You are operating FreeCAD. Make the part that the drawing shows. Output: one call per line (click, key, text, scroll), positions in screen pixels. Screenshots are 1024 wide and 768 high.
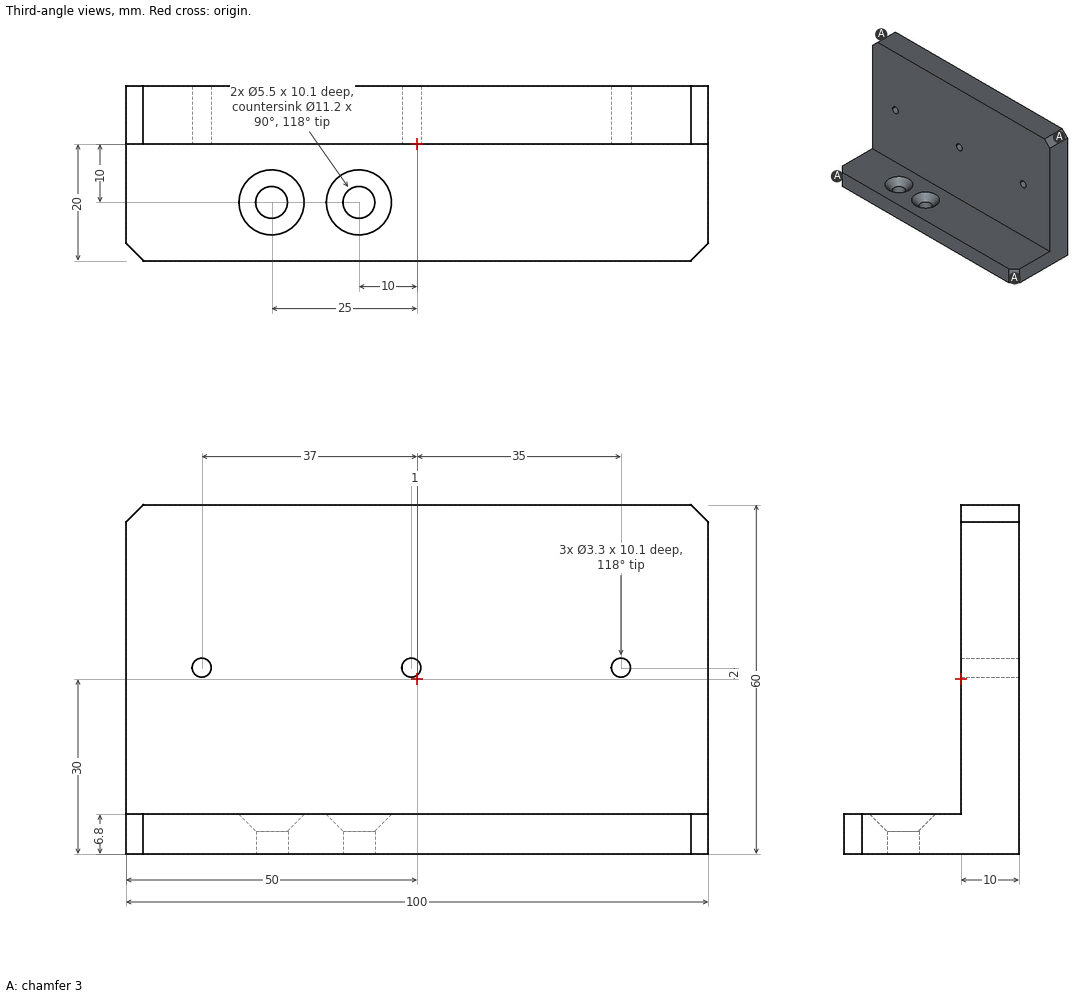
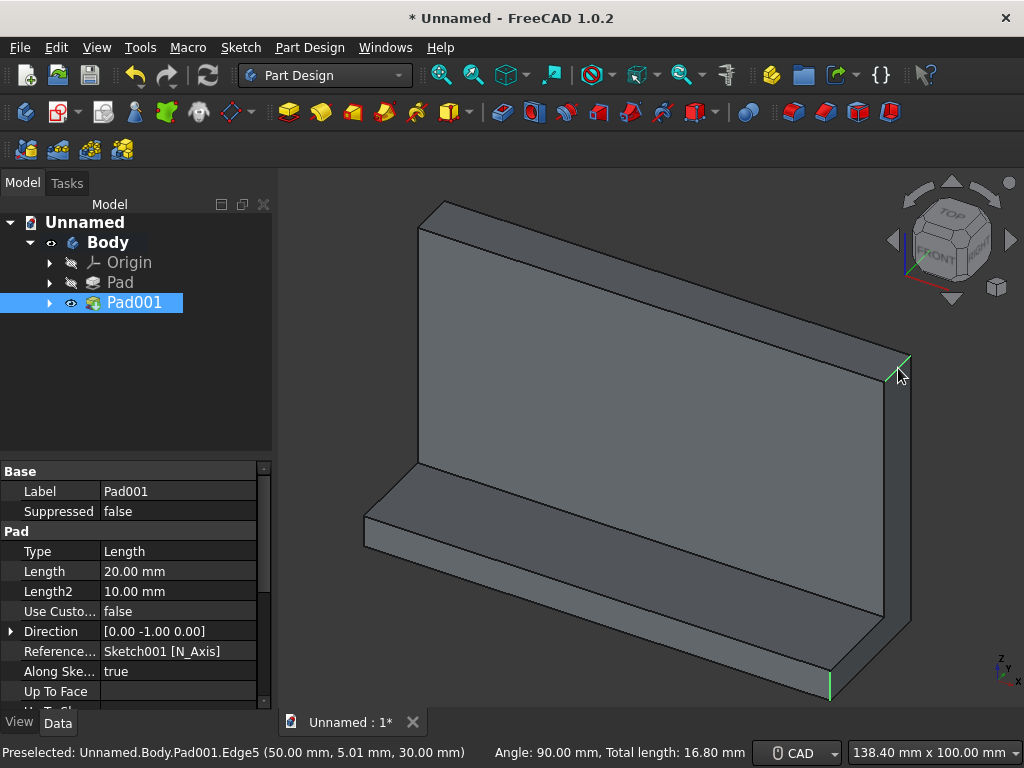
key(0)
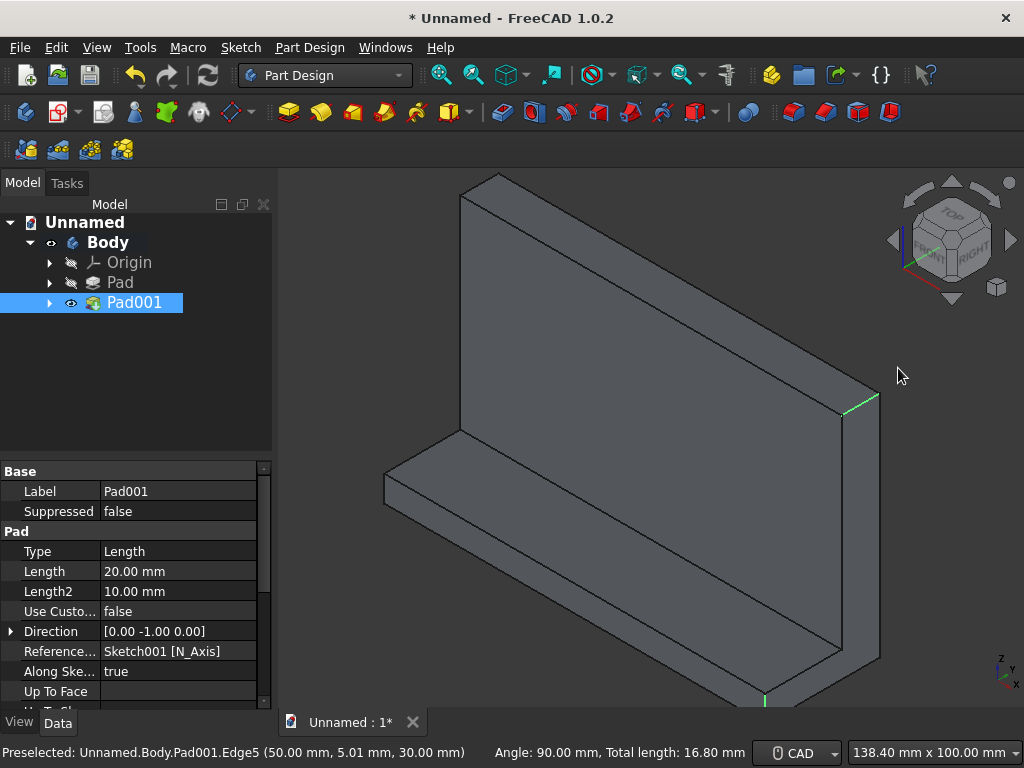
key(v)
key(f)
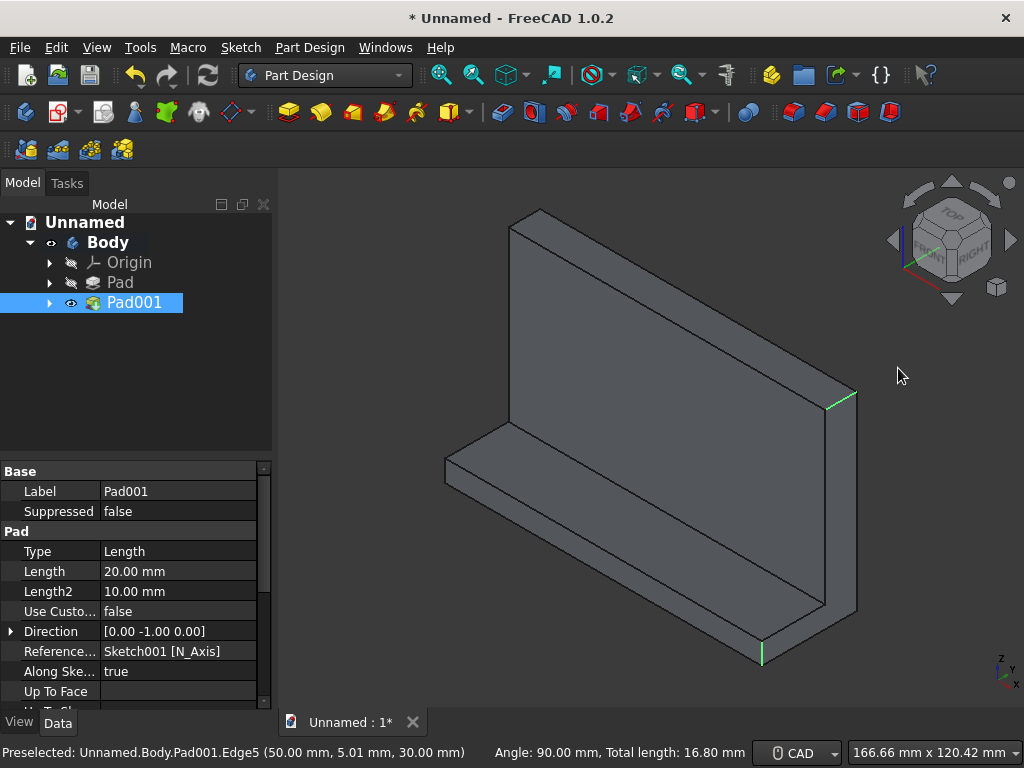
key(2)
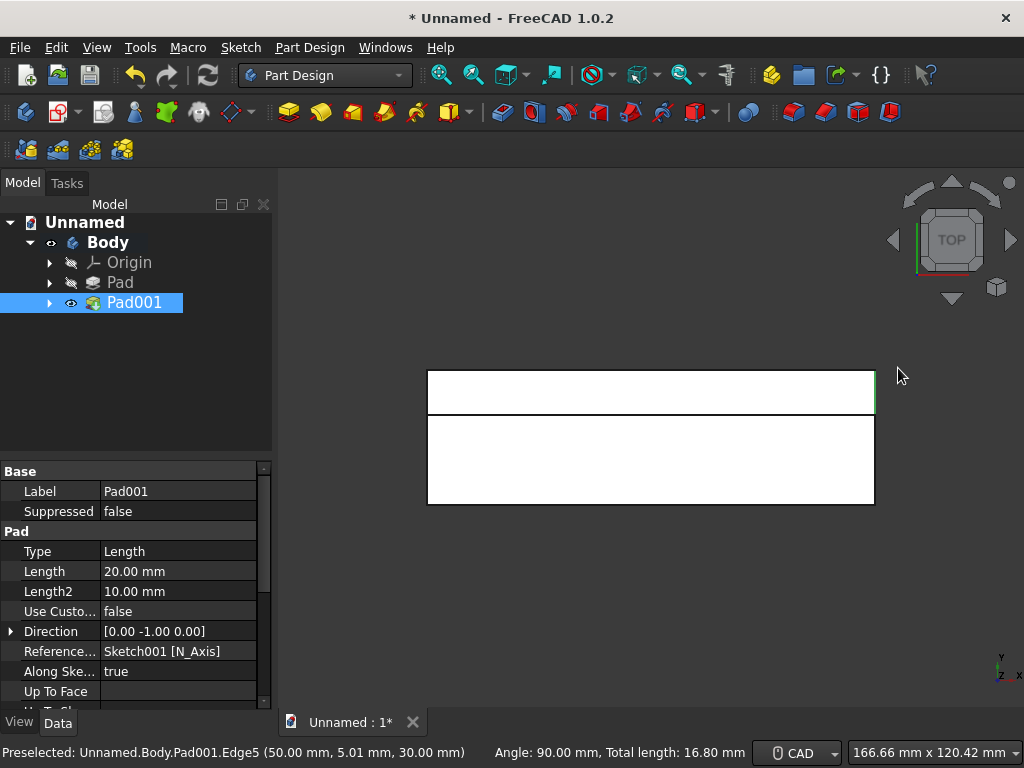
click(427, 392, ctrl)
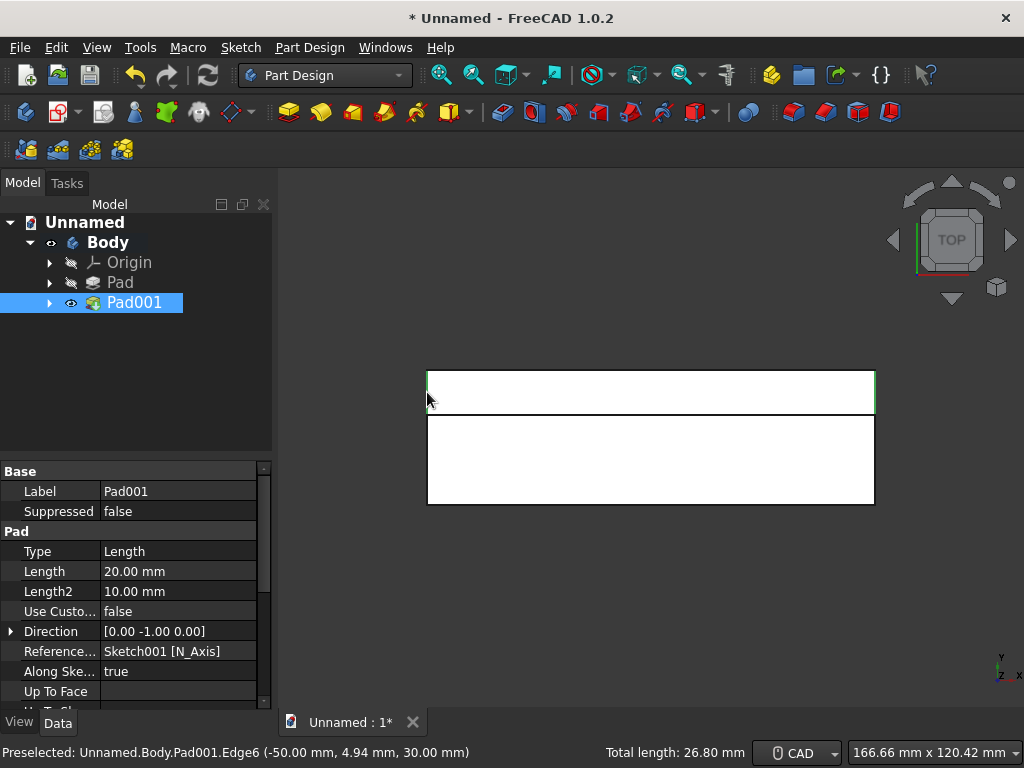
key(1)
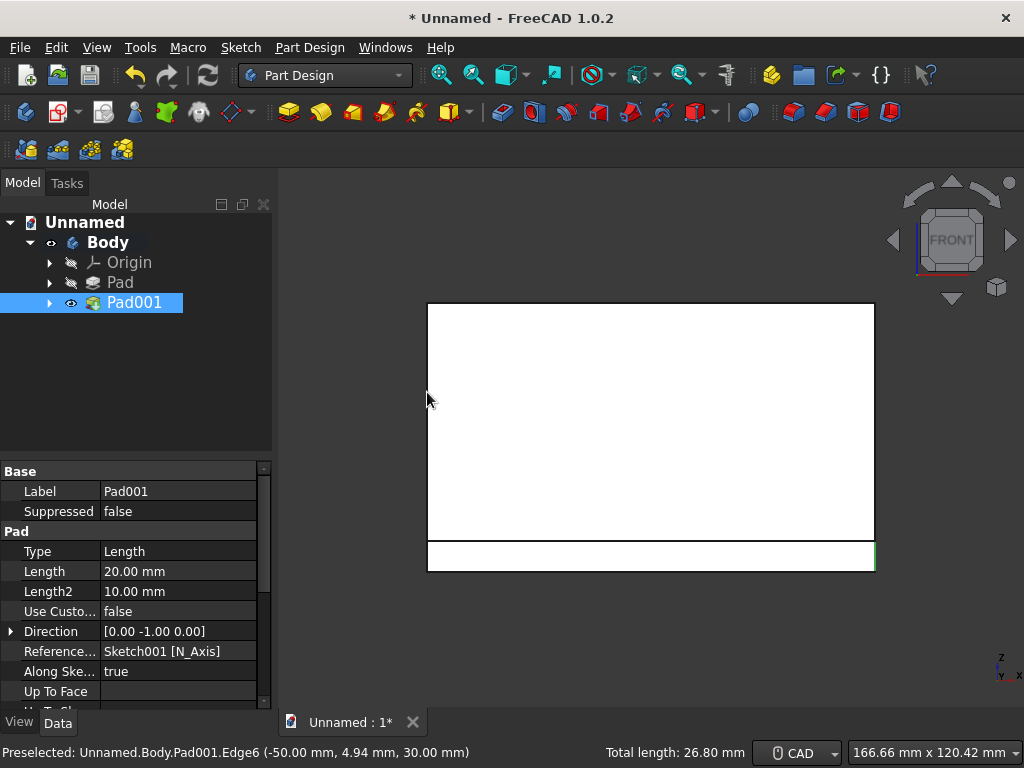
click(427, 556, ctrl)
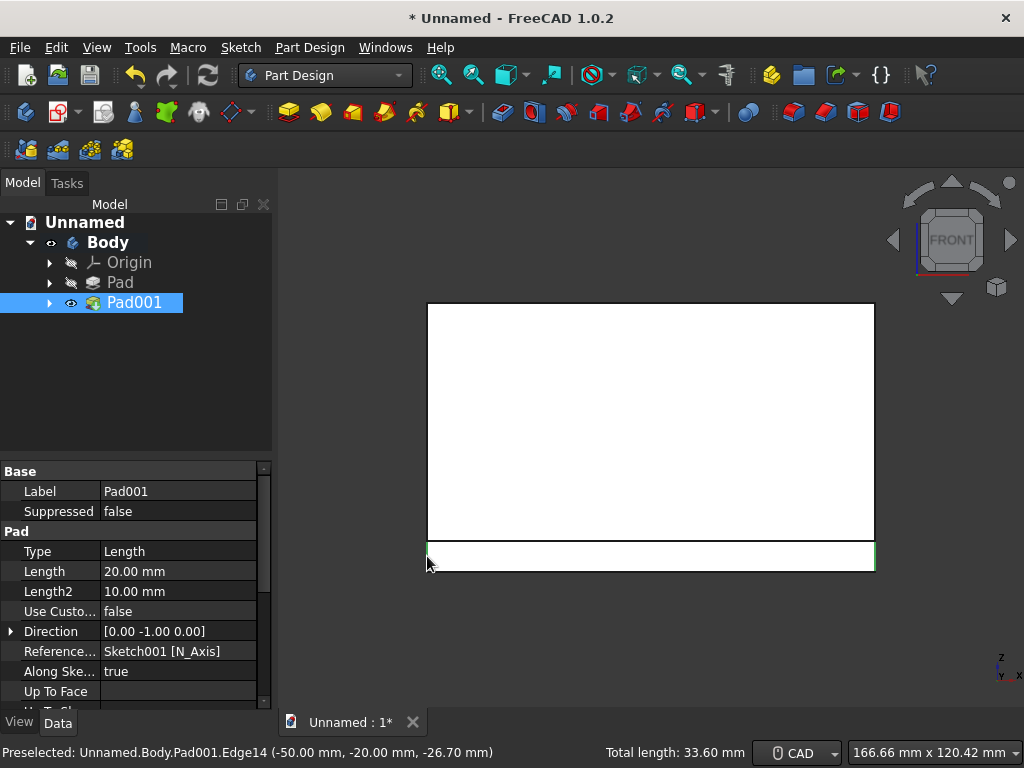
click(826, 112)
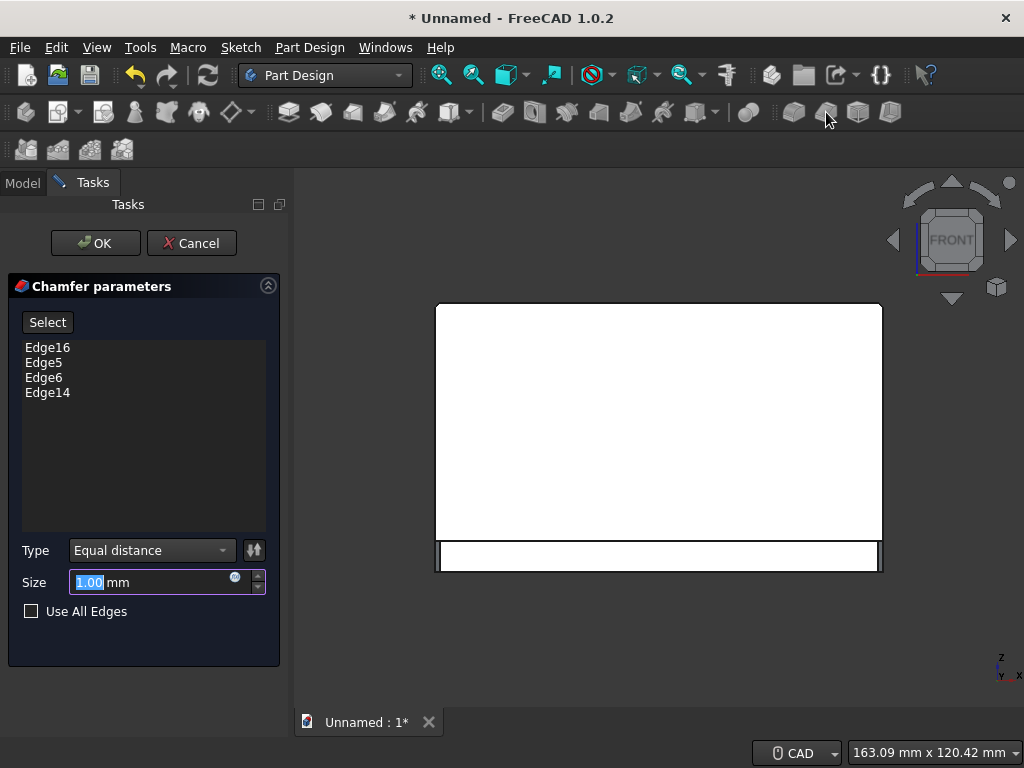
text(3)
key(Tab)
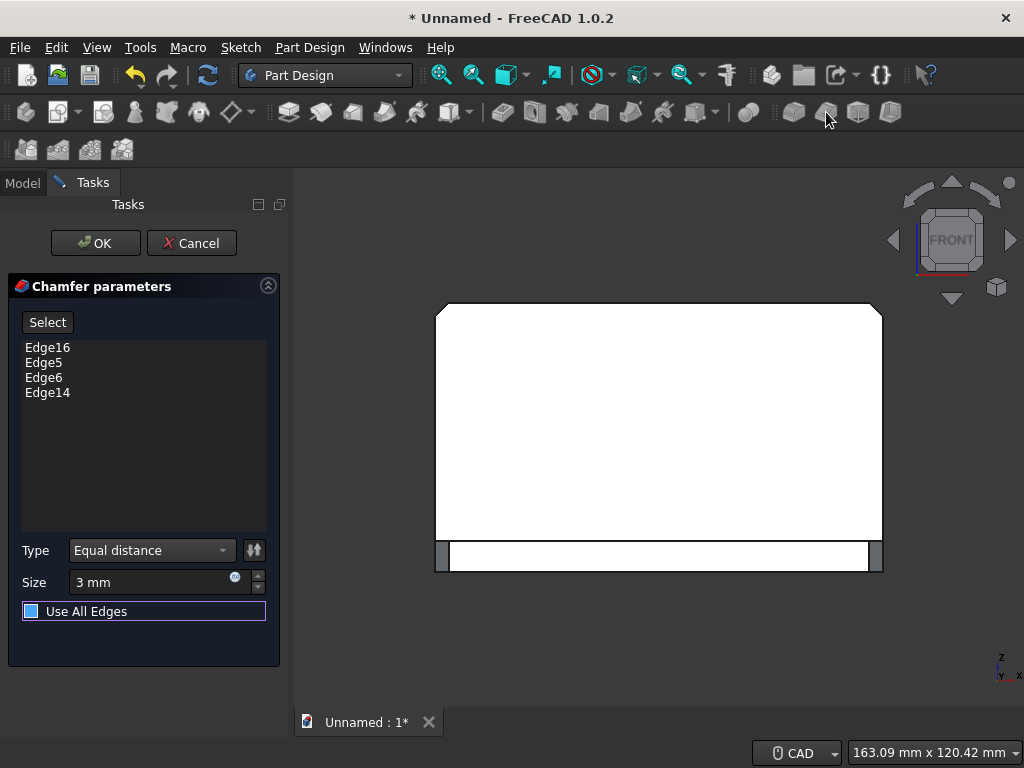
click(96, 243)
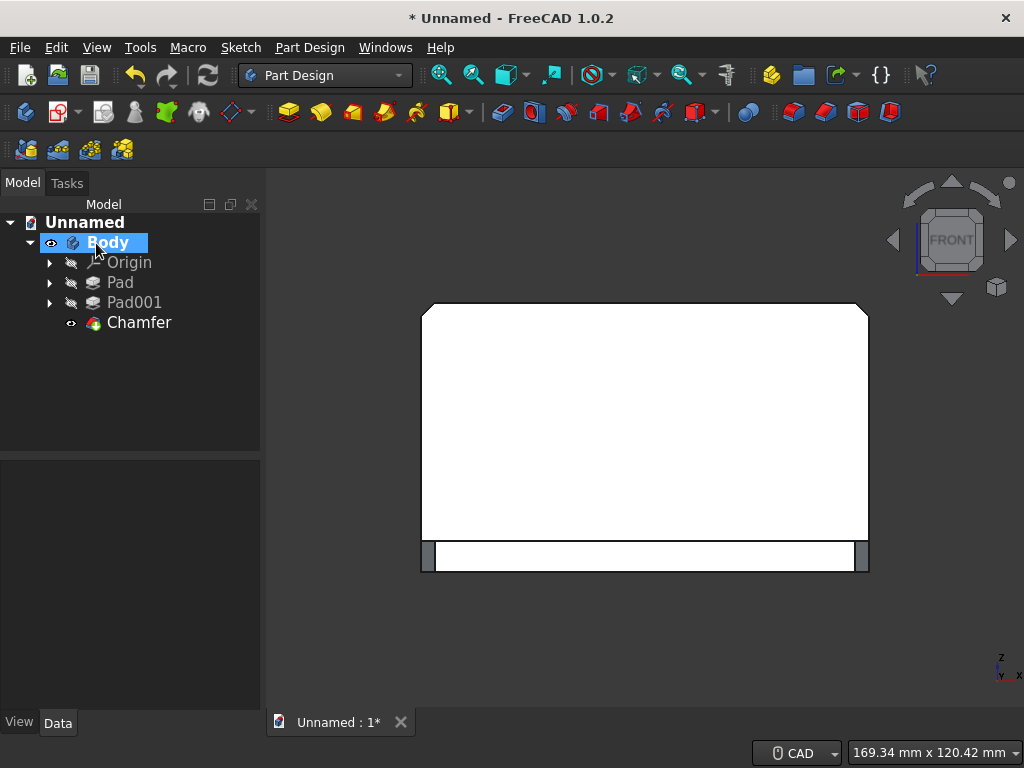
key(4)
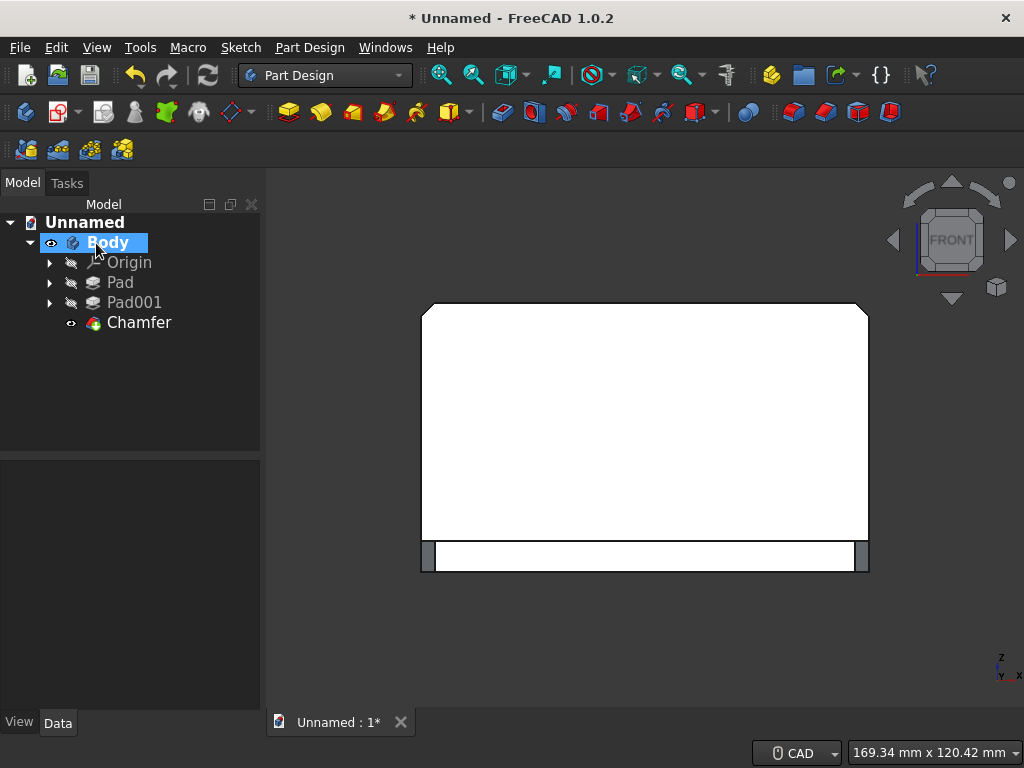
click(581, 437)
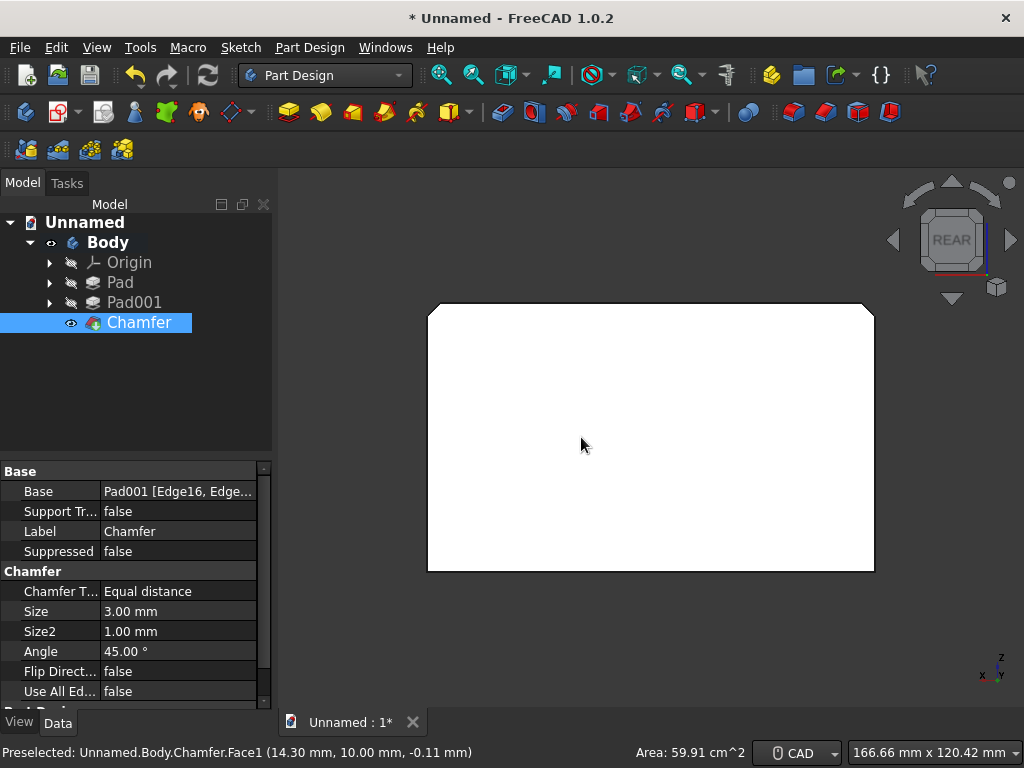
click(58, 112)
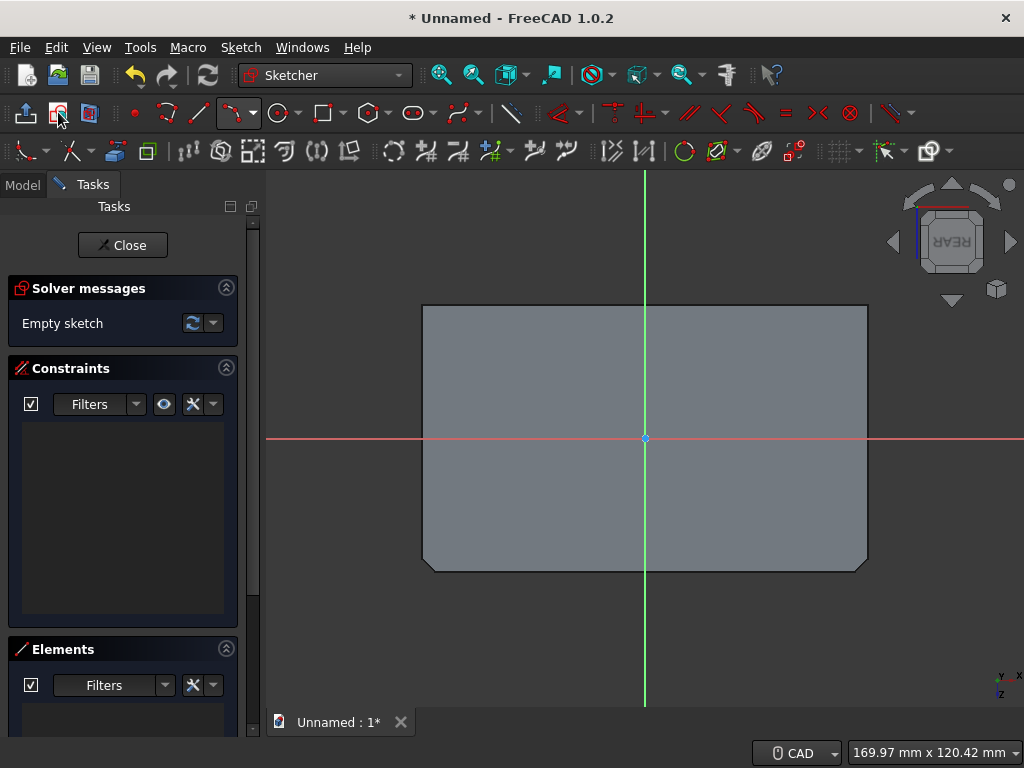
key(g)
key(c)